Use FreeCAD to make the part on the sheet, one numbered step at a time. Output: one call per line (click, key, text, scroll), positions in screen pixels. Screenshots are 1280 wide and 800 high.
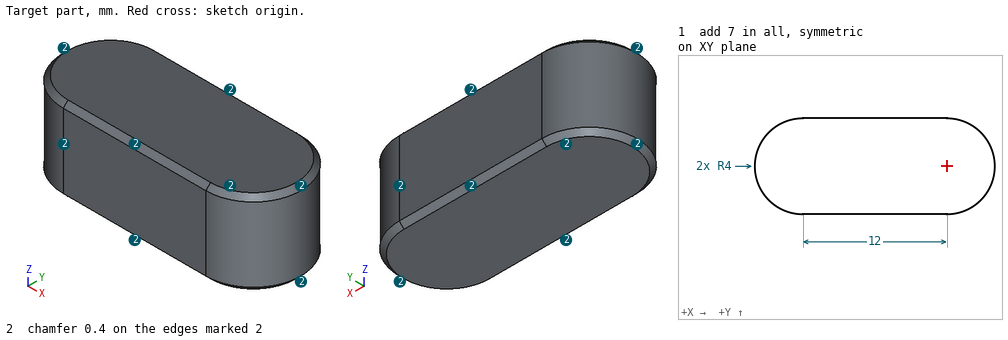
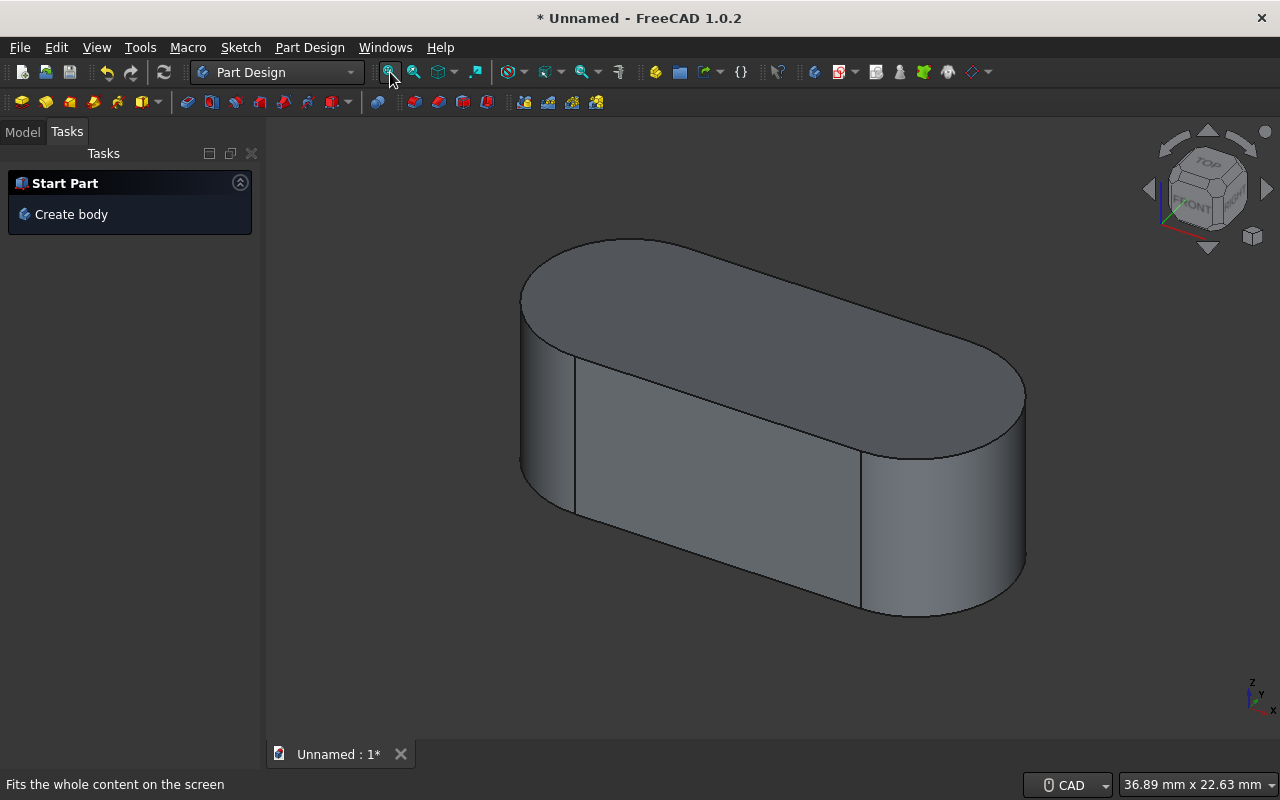
click(909, 393)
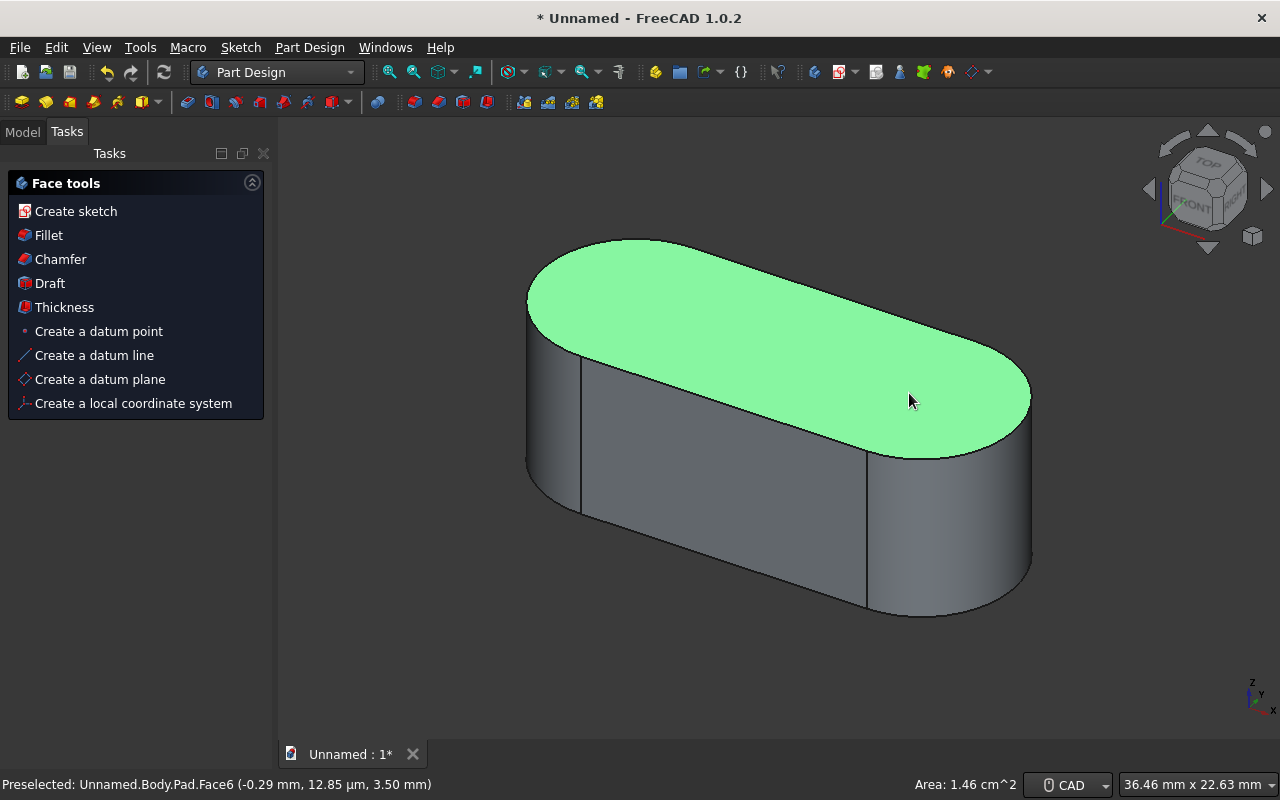
key(0)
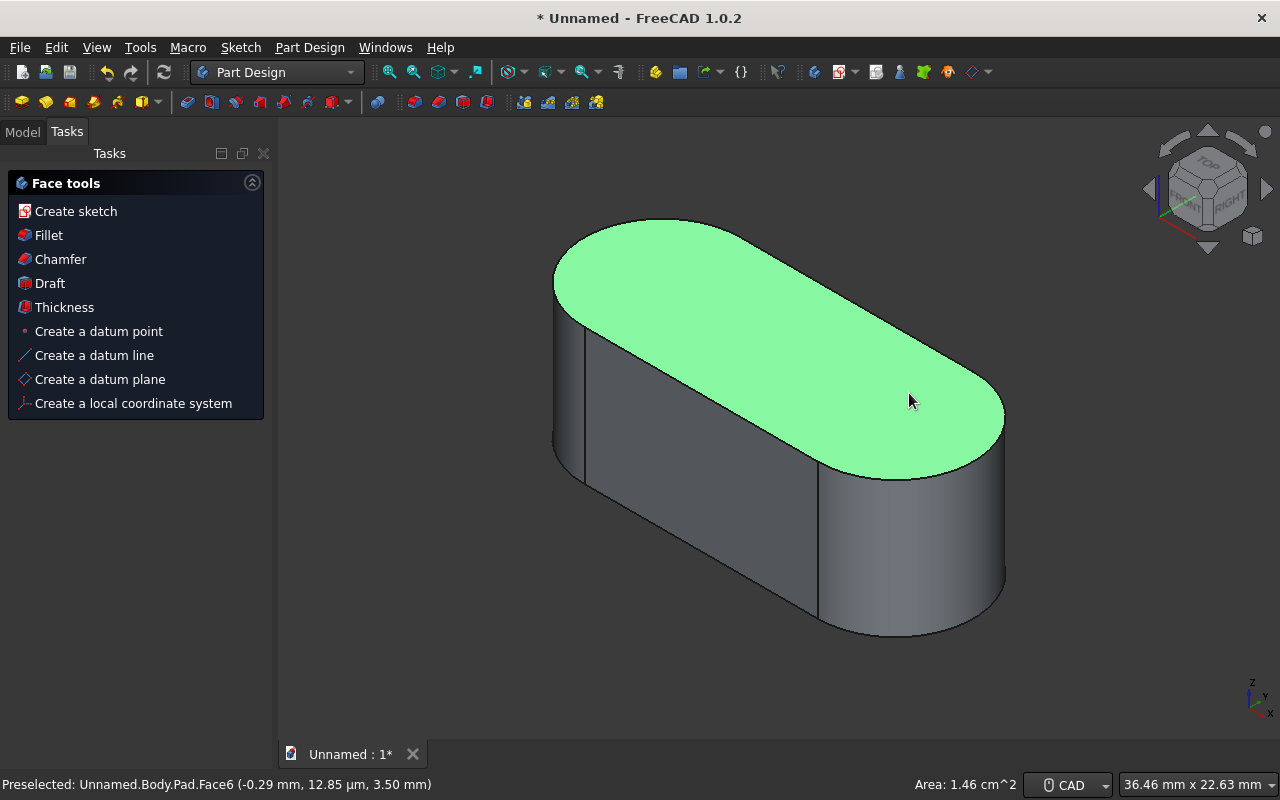
key(2)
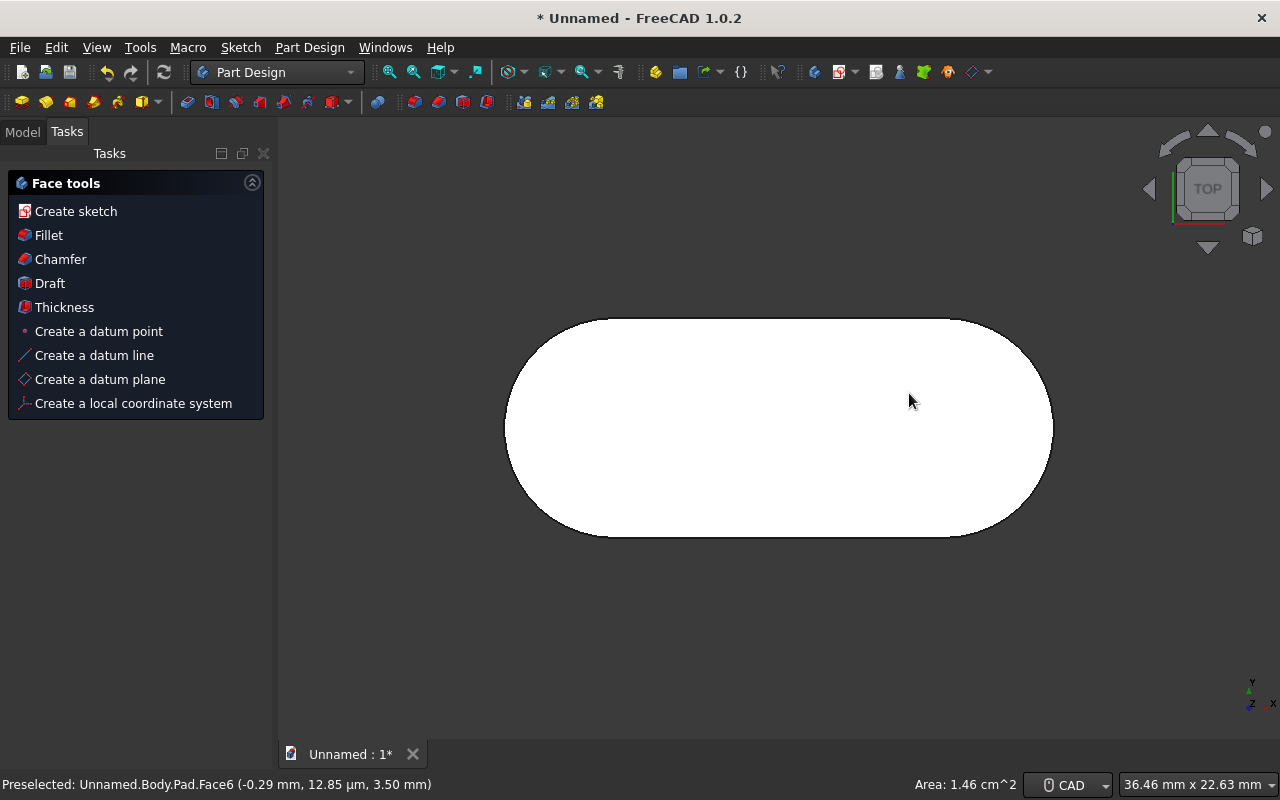
key(1)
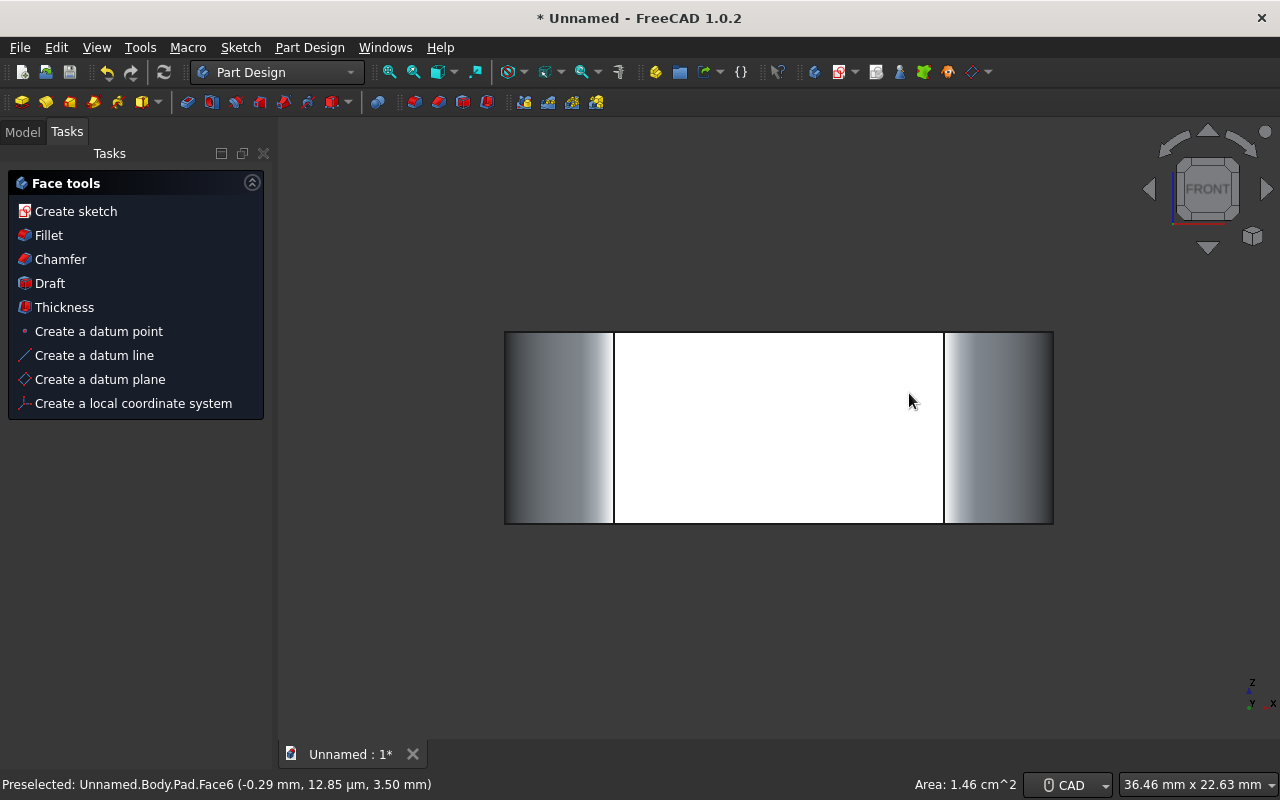
key(3)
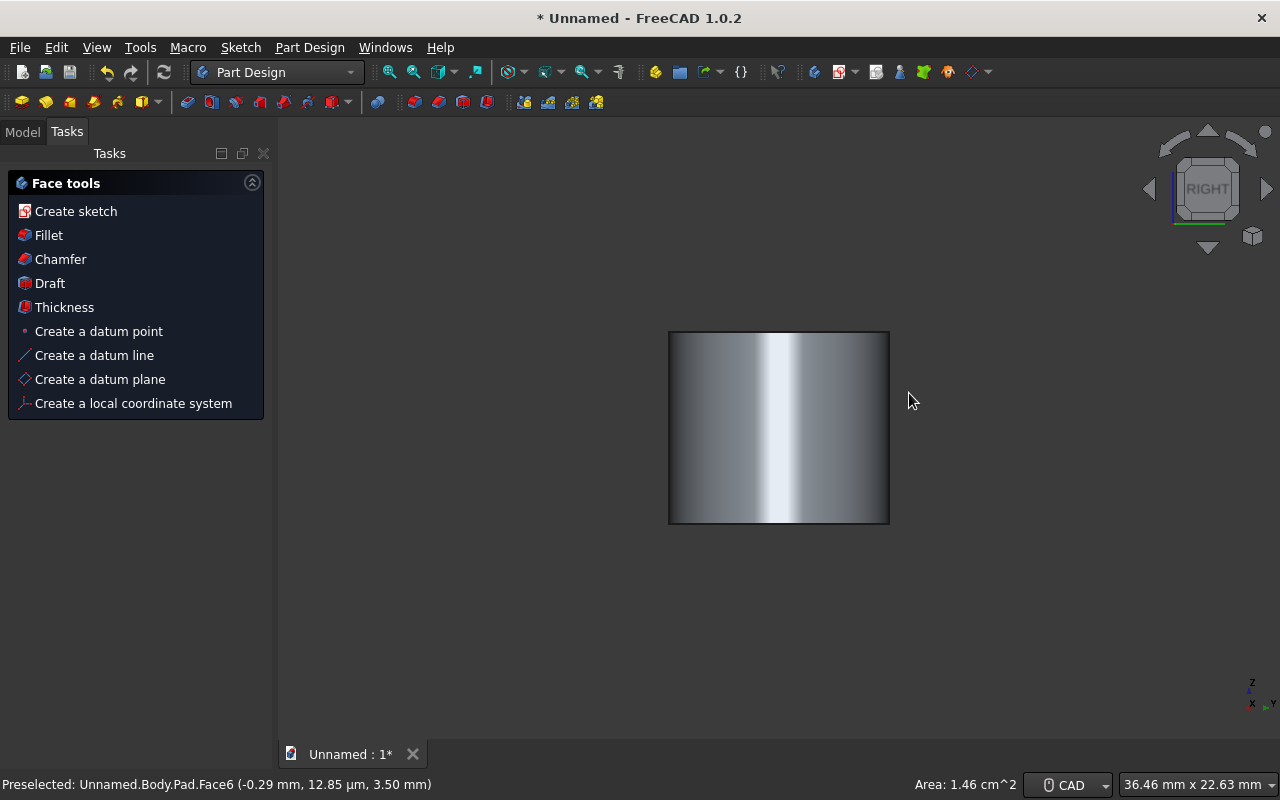
click(390, 72)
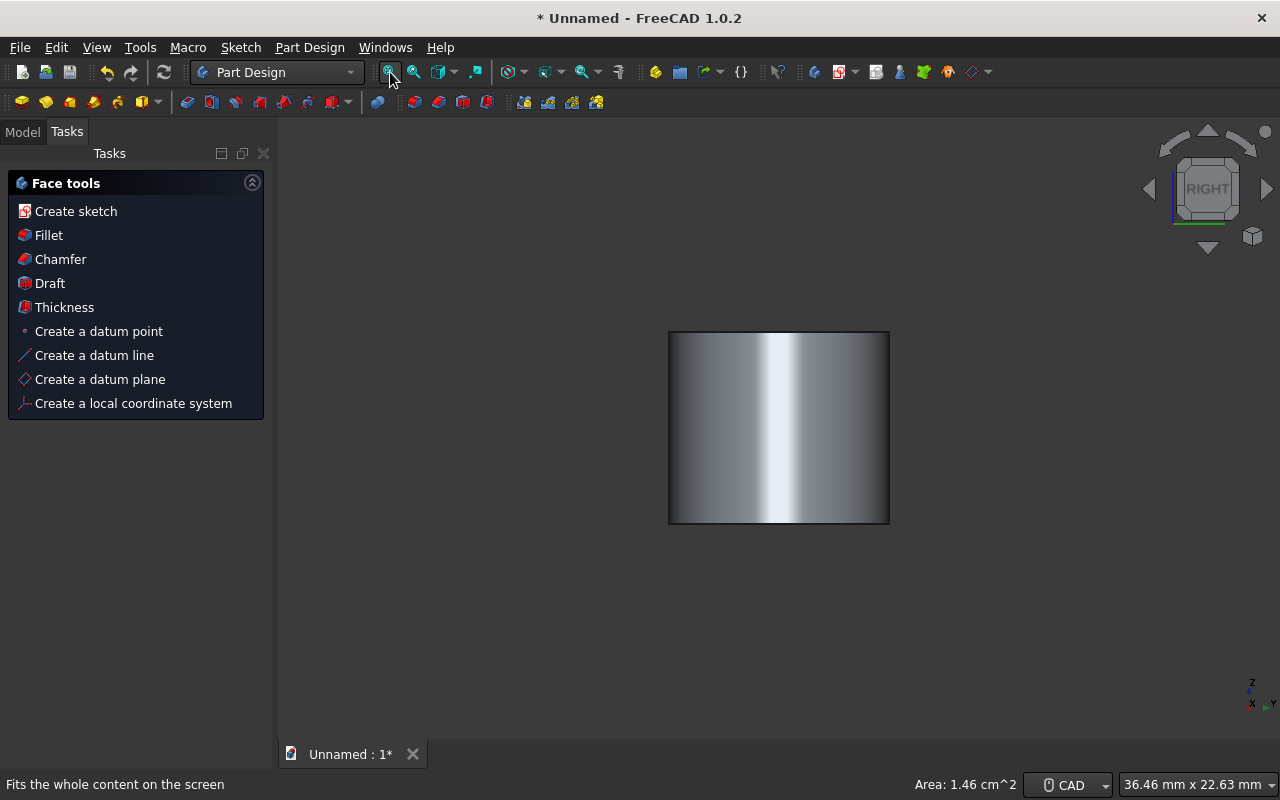
key(5)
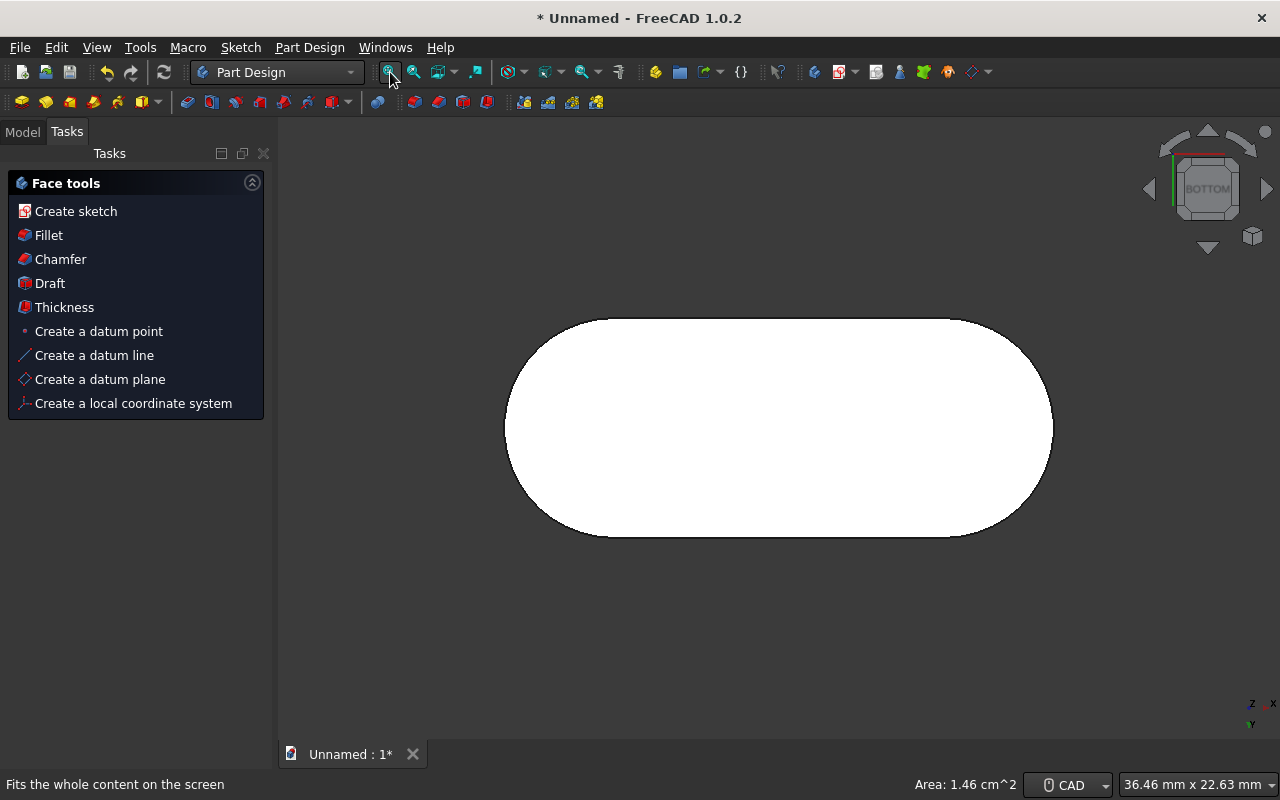
click(936, 427, ctrl)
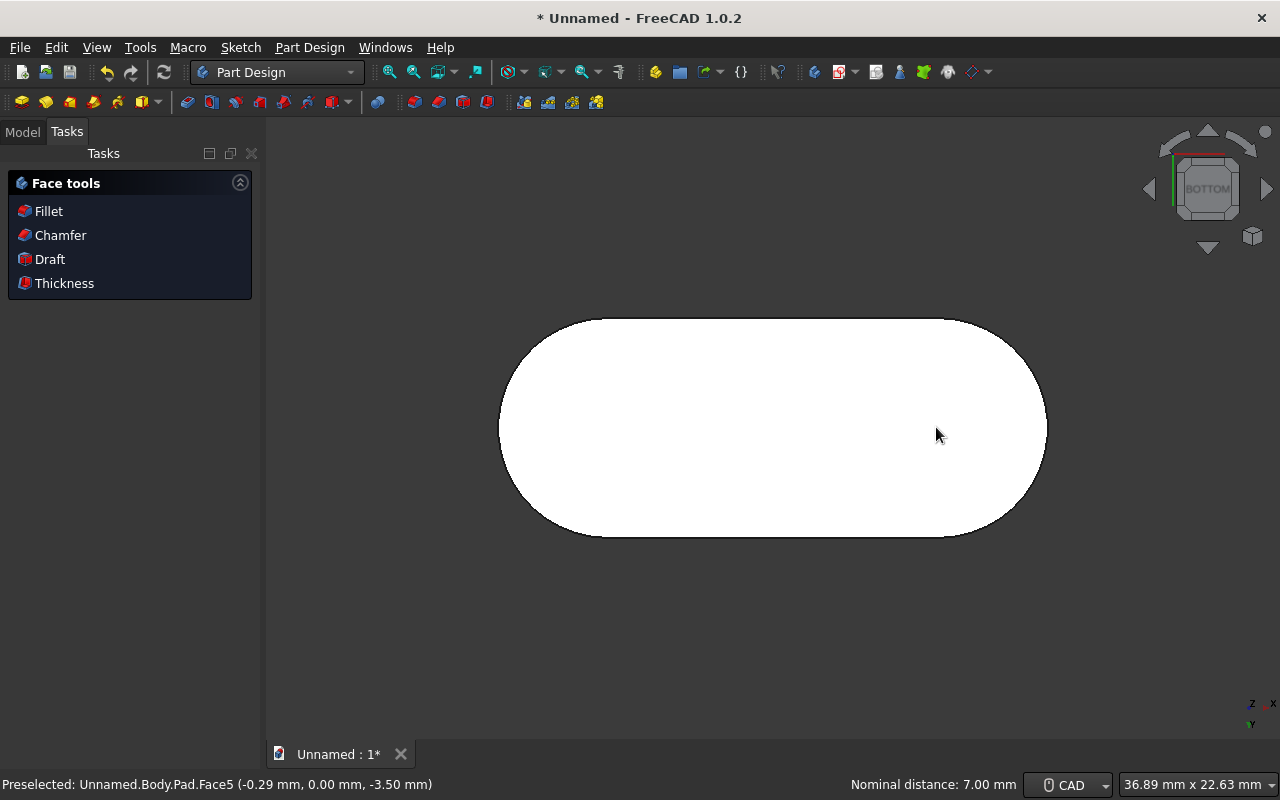
click(440, 102)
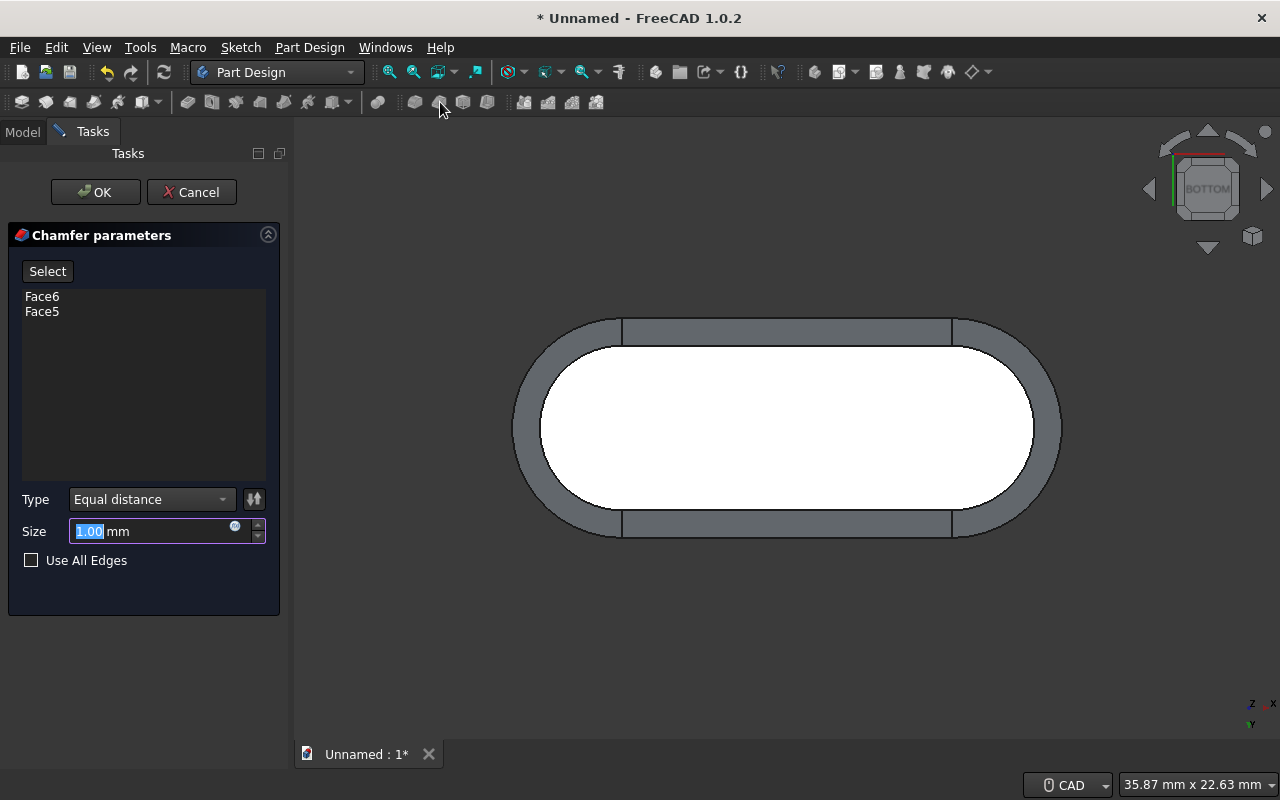
text(0.4)
key(Tab)